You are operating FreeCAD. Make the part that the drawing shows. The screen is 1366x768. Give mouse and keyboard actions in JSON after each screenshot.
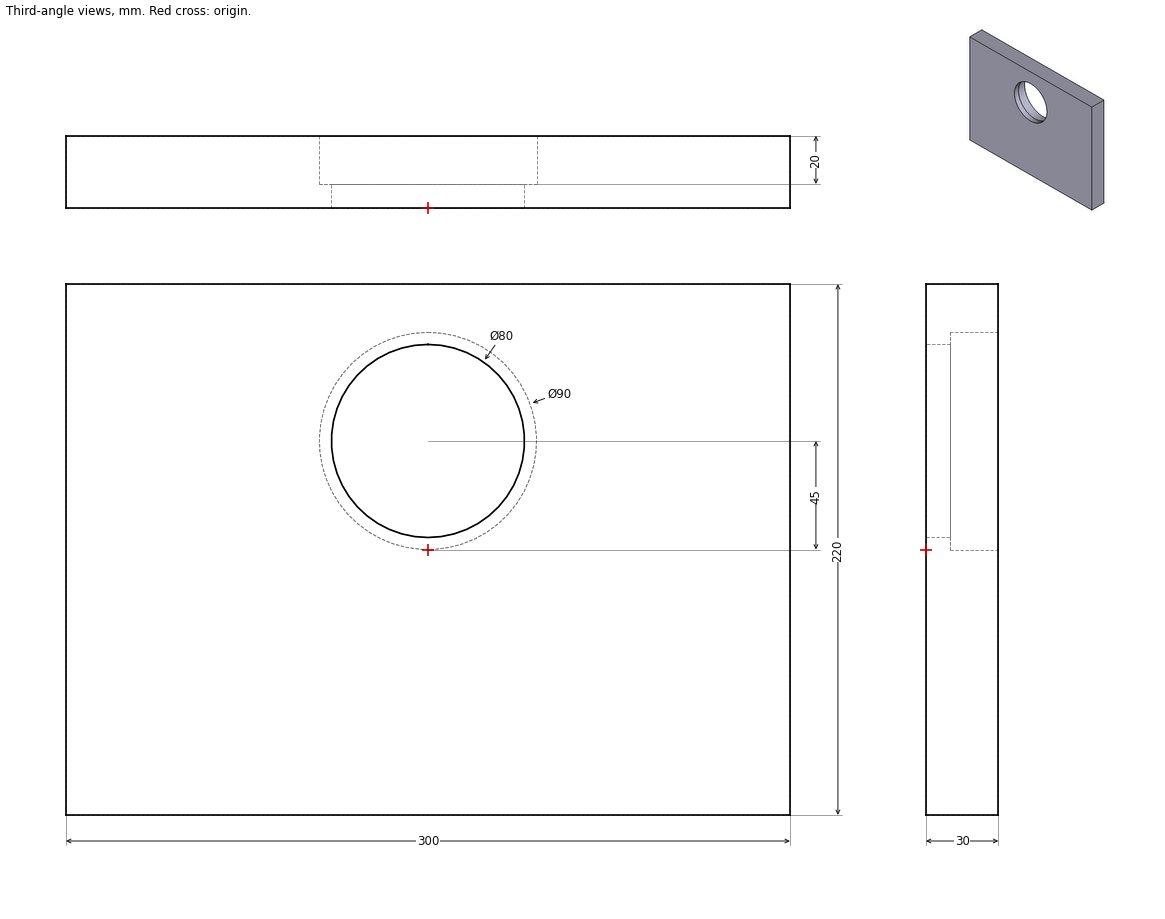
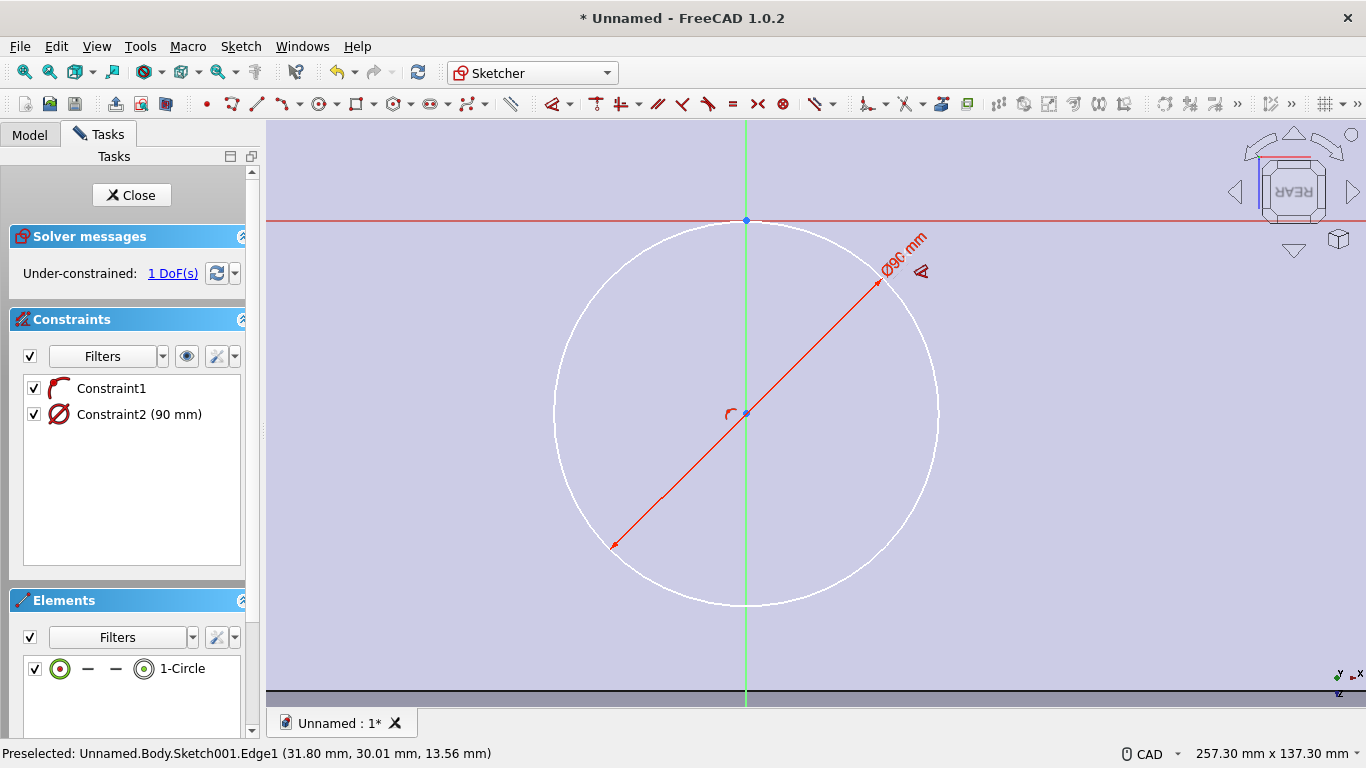
{"action": "left_click", "coordinate": [746, 414]}
{"action": "left_click", "coordinate": [780, 317]}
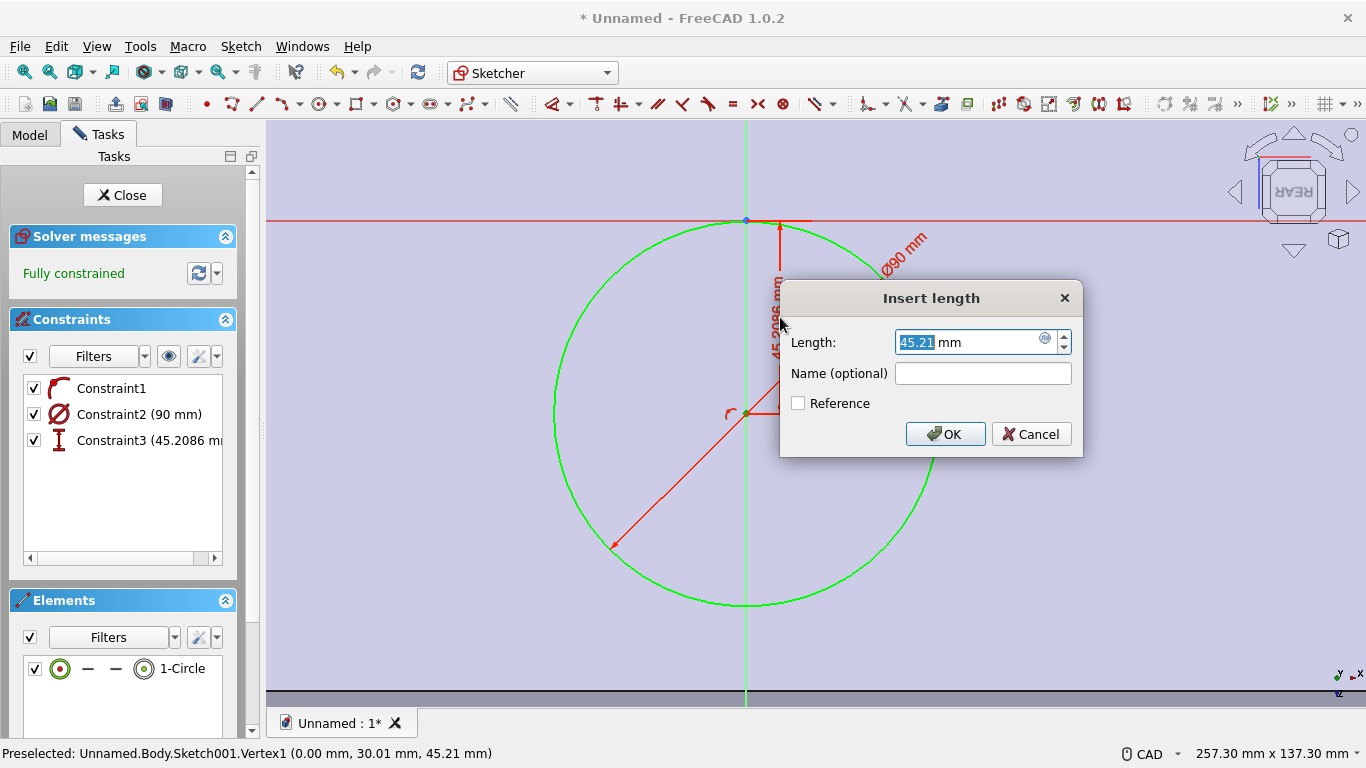
{"action": "type", "text": "45"}
{"action": "key", "text": "Return"}
{"action": "key", "text": "Escape"}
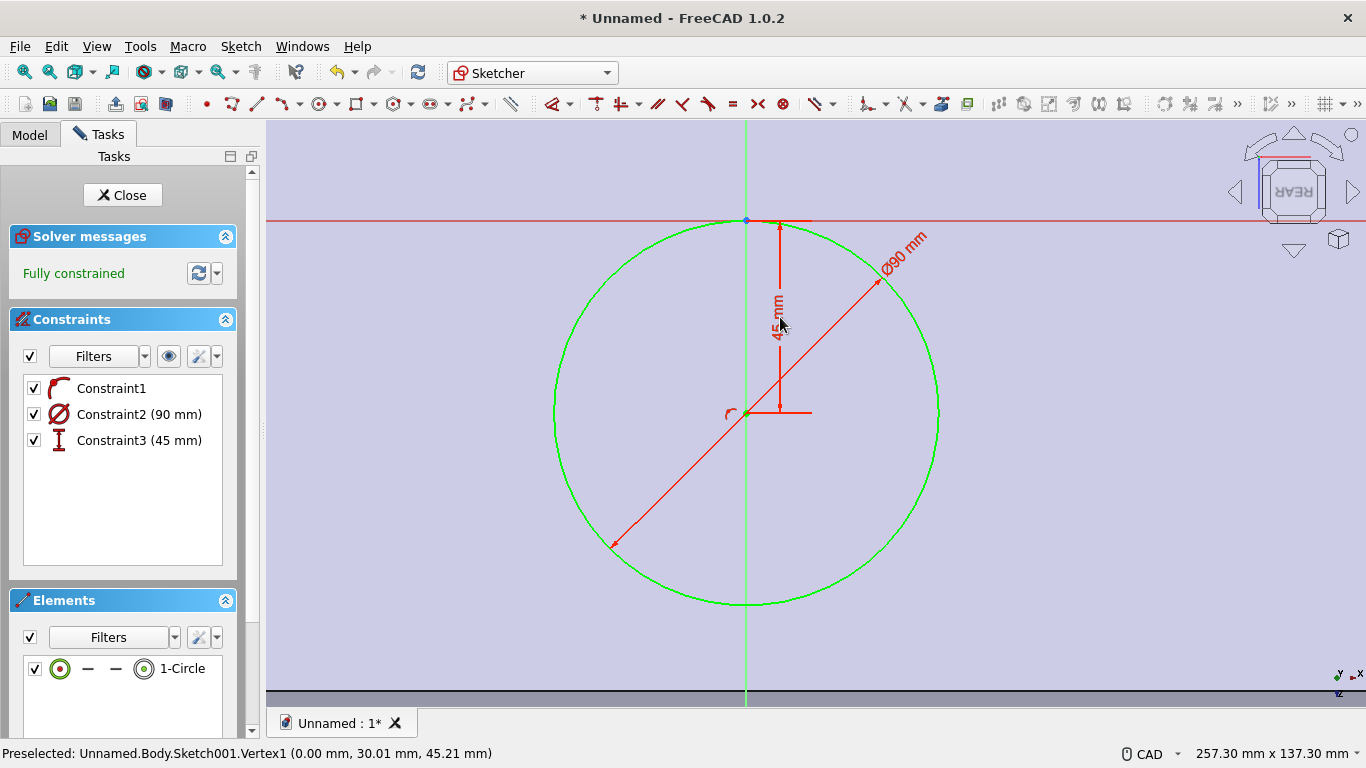
{"action": "left_click", "coordinate": [123, 195]}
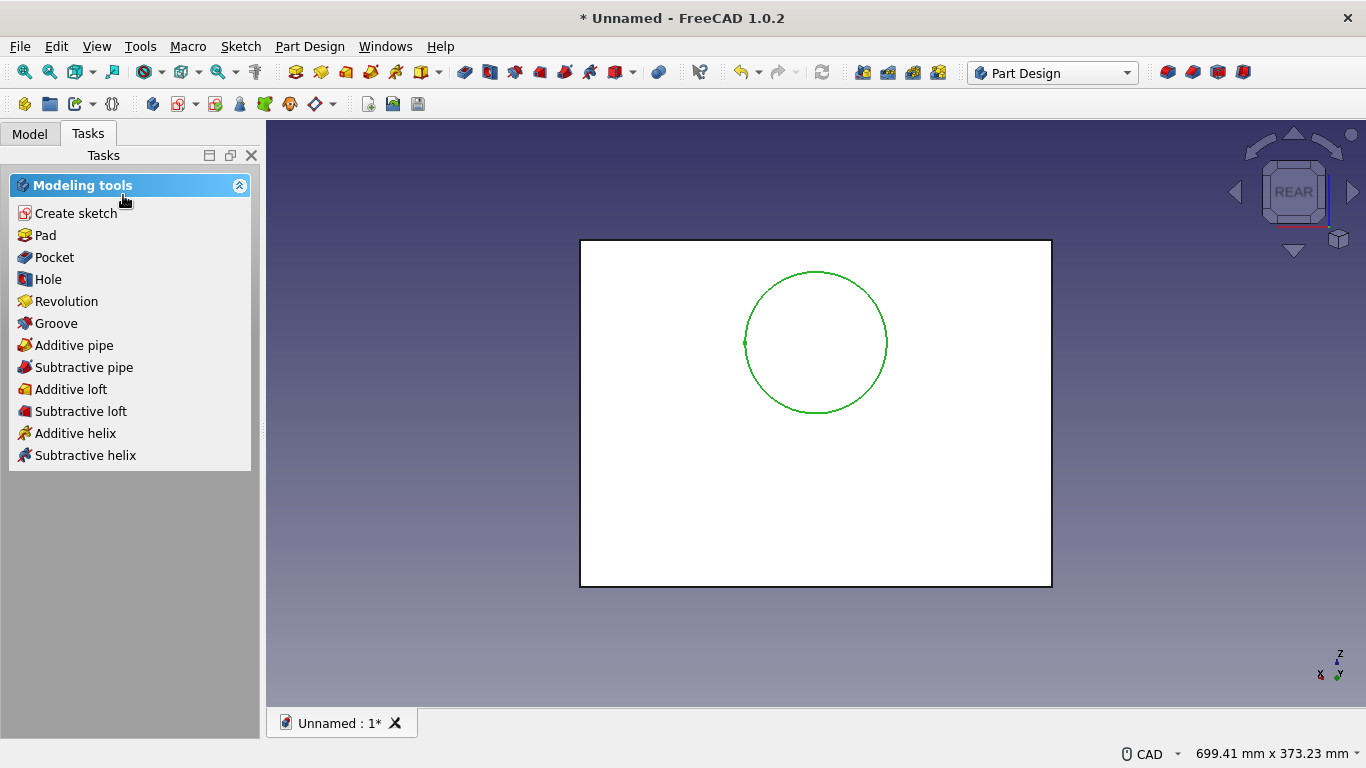
{"action": "left_click", "coordinate": [465, 72]}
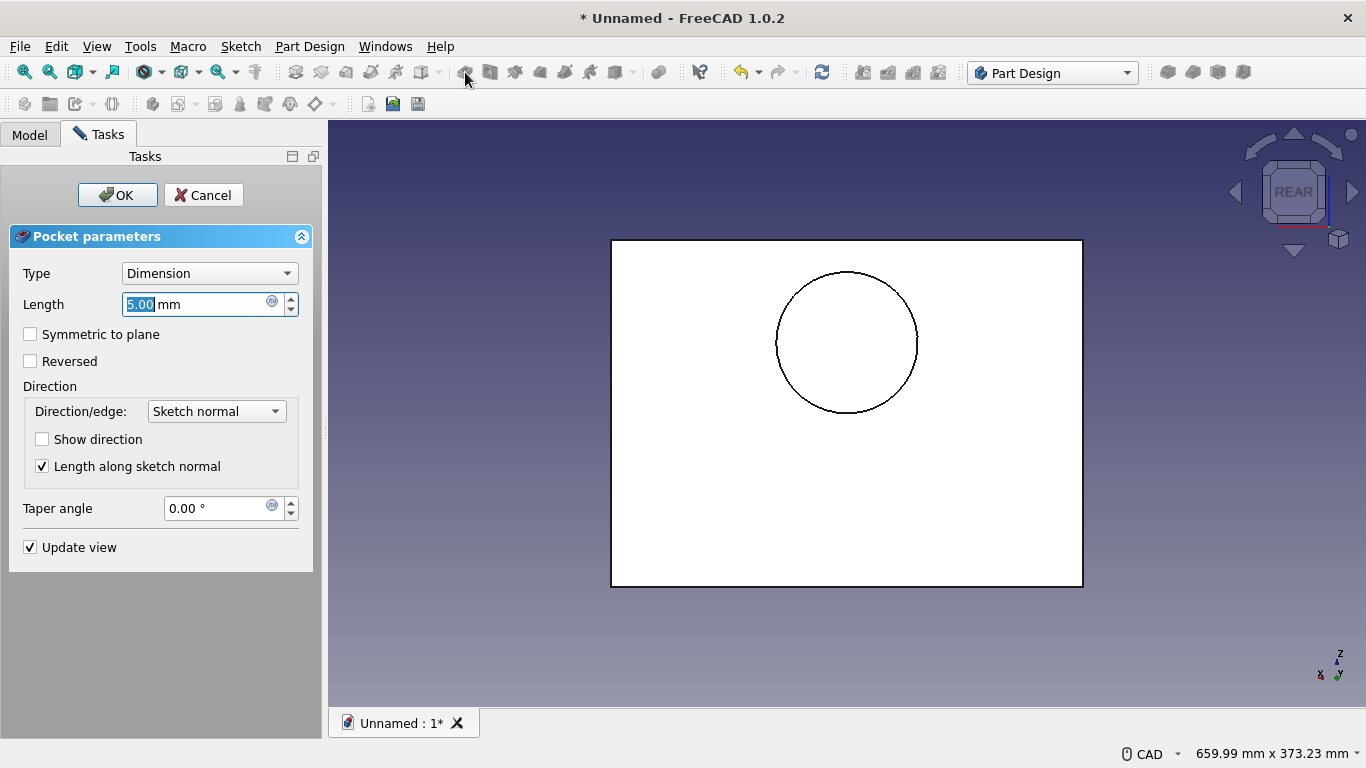
{"action": "type", "text": "20"}
{"action": "key", "text": "Tab"}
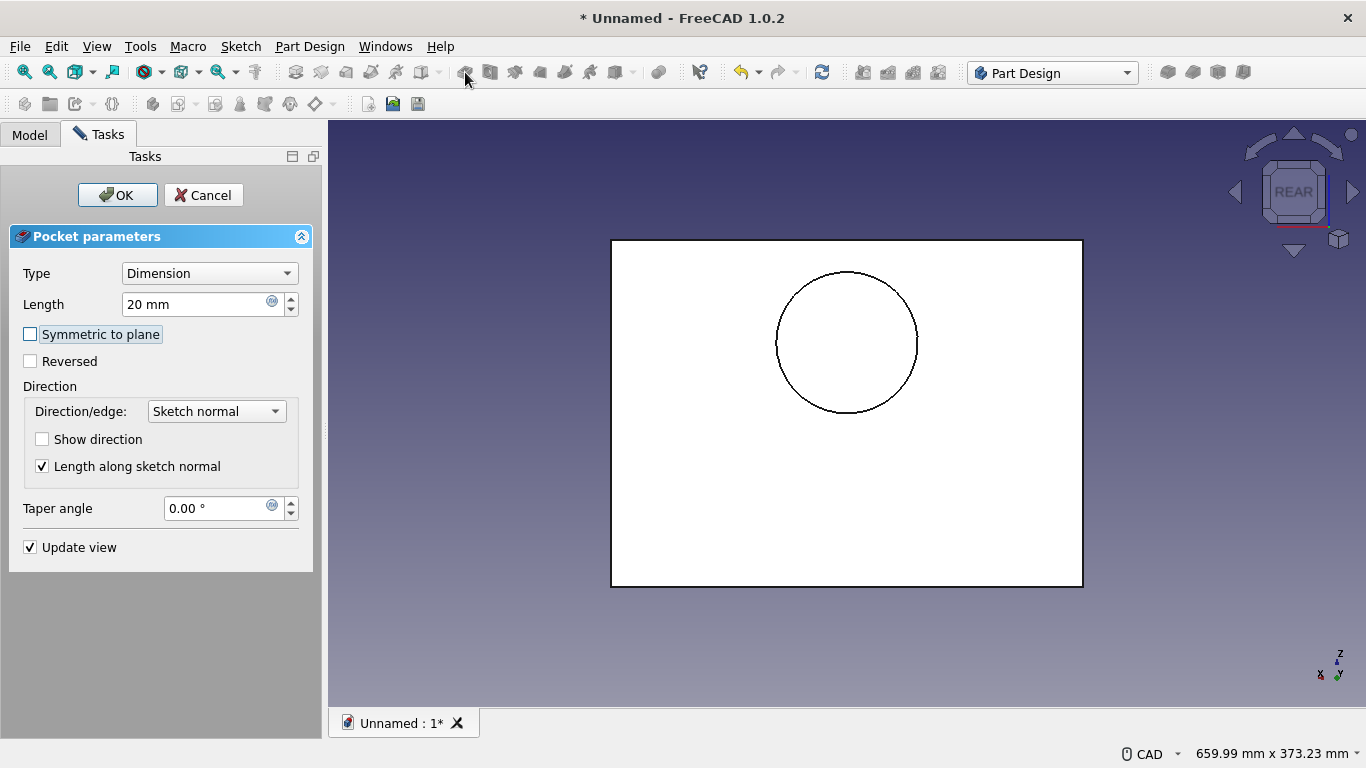
{"action": "left_click", "coordinate": [118, 195]}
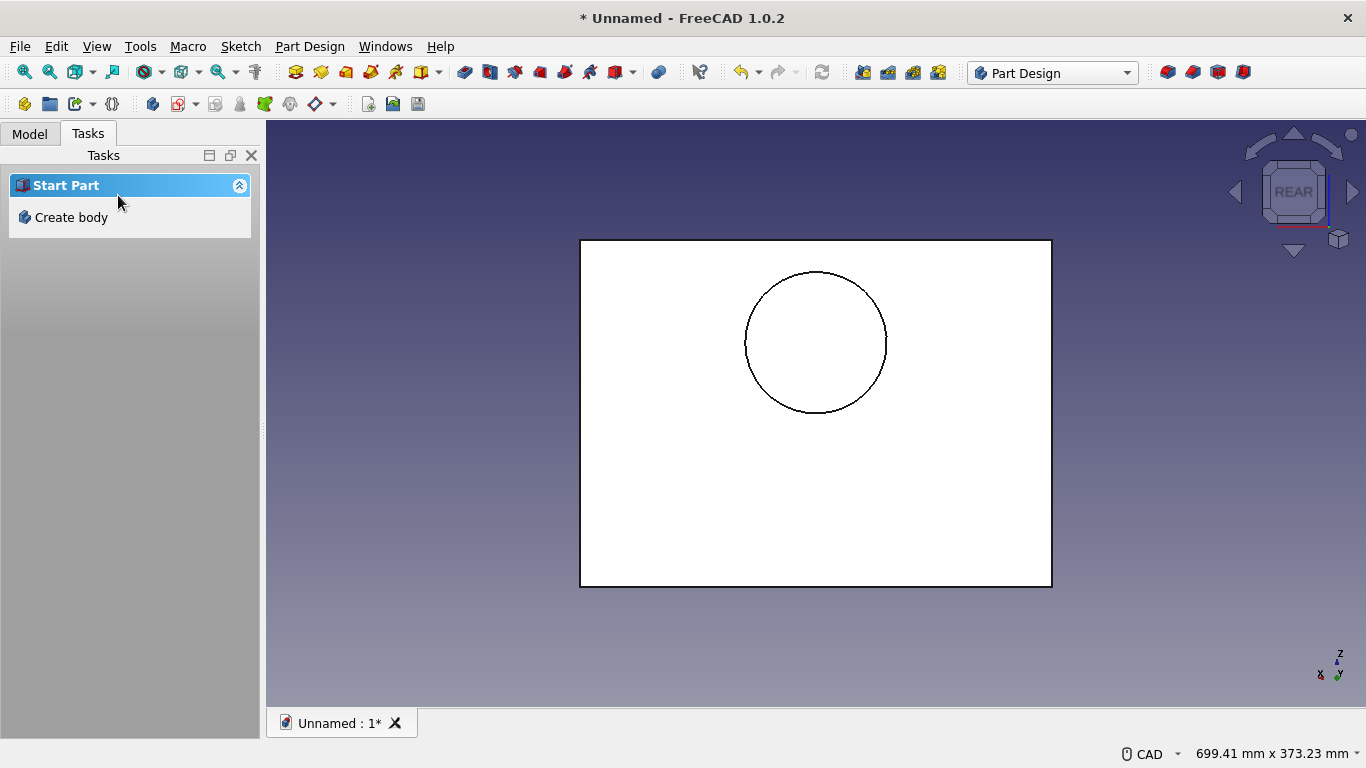
{"action": "left_click", "coordinate": [951, 462]}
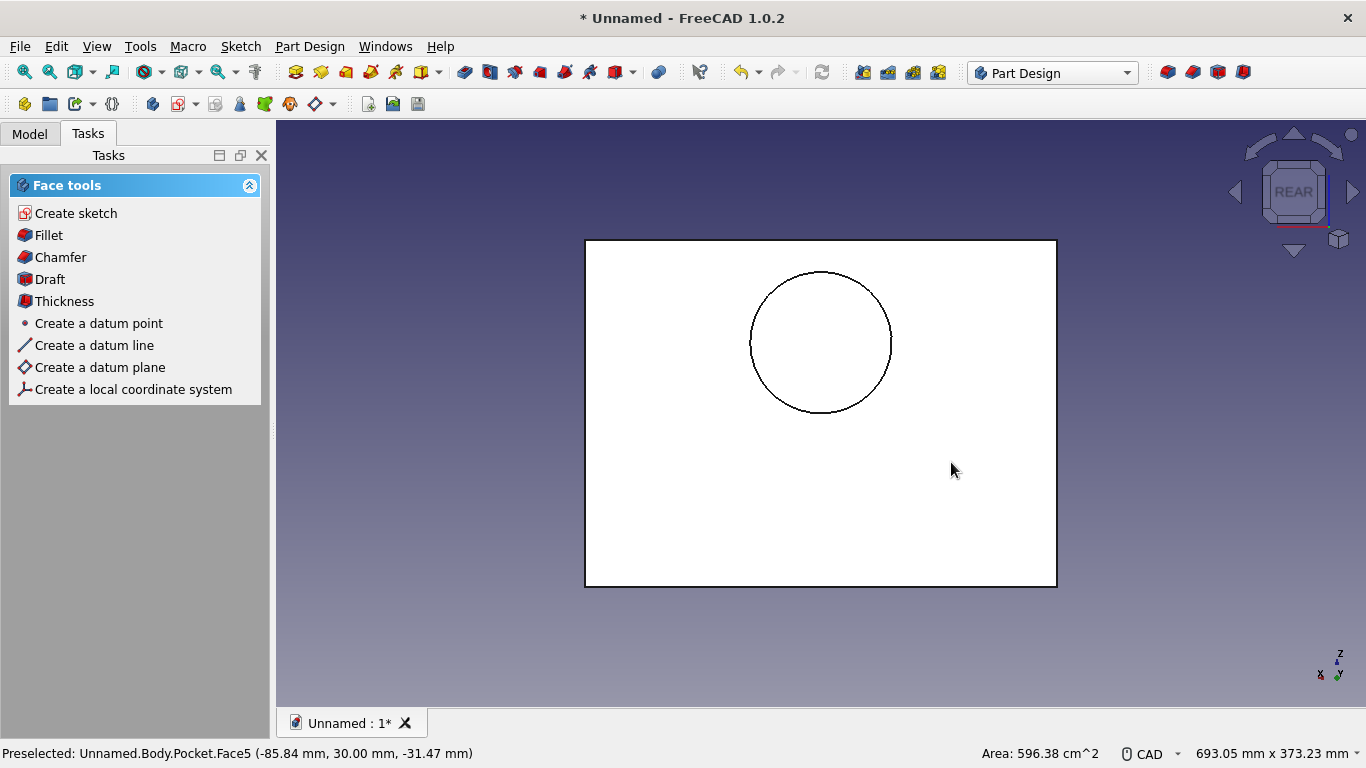
{"action": "left_click", "coordinate": [178, 104]}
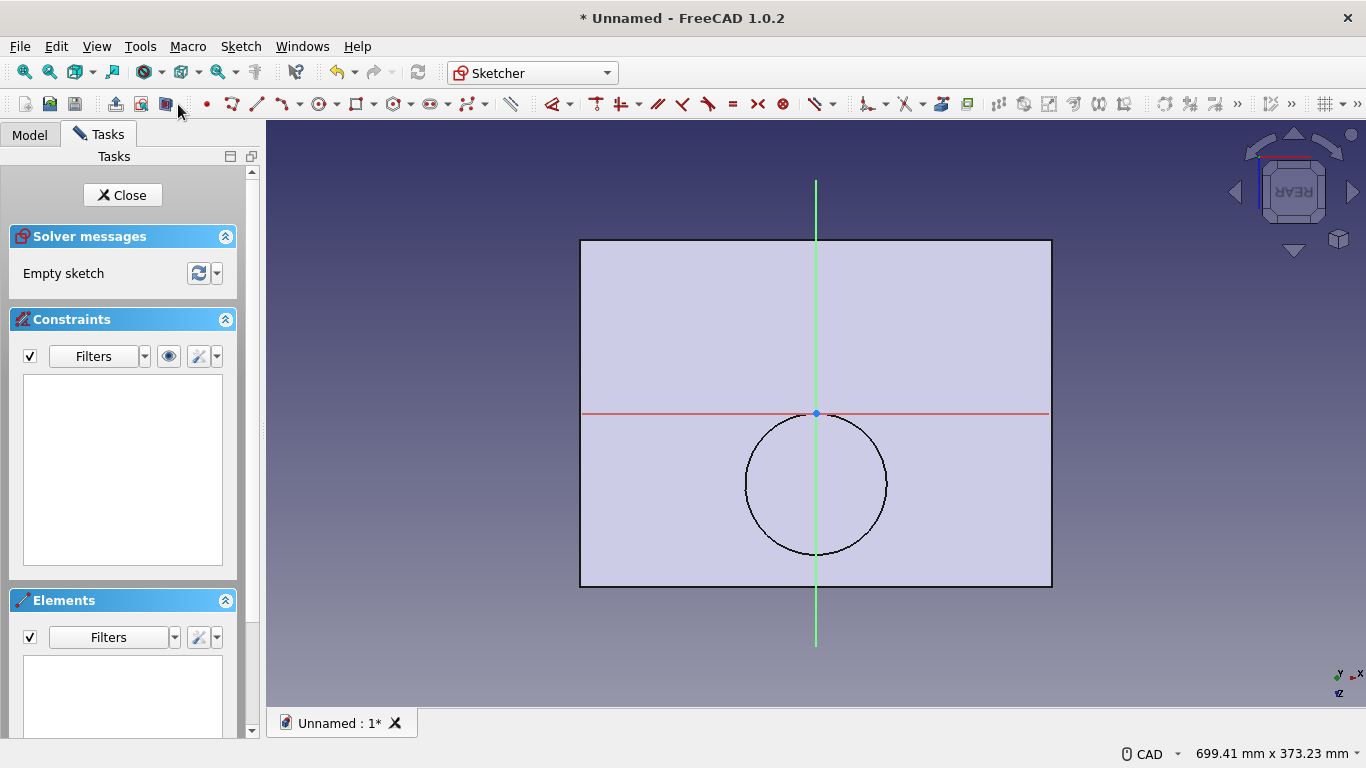
{"action": "scroll", "coordinate": [856, 519], "scroll_direction": "up", "scroll_amount": 5}